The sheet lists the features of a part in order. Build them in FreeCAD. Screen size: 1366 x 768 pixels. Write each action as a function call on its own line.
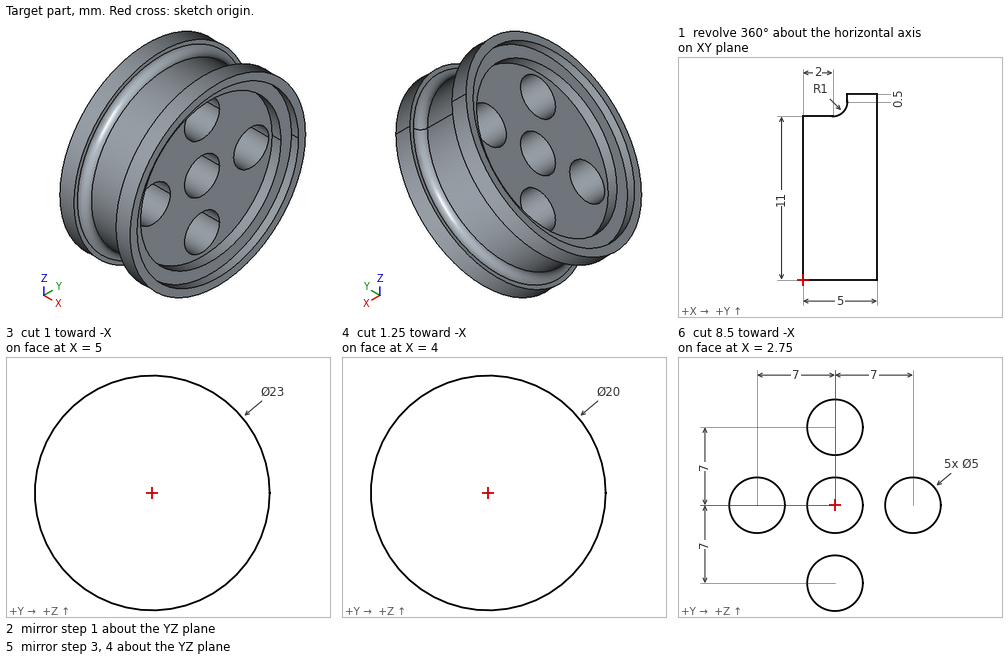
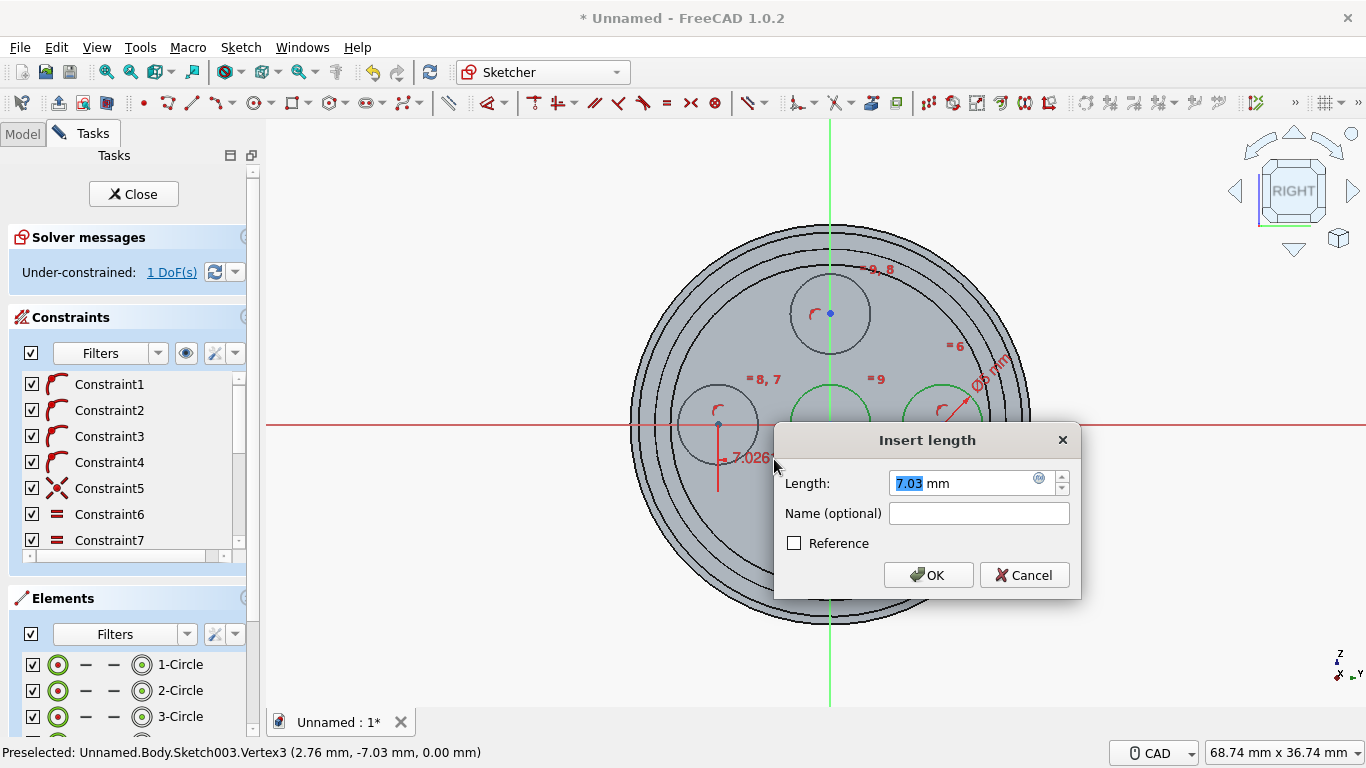
text(7)
key(Return)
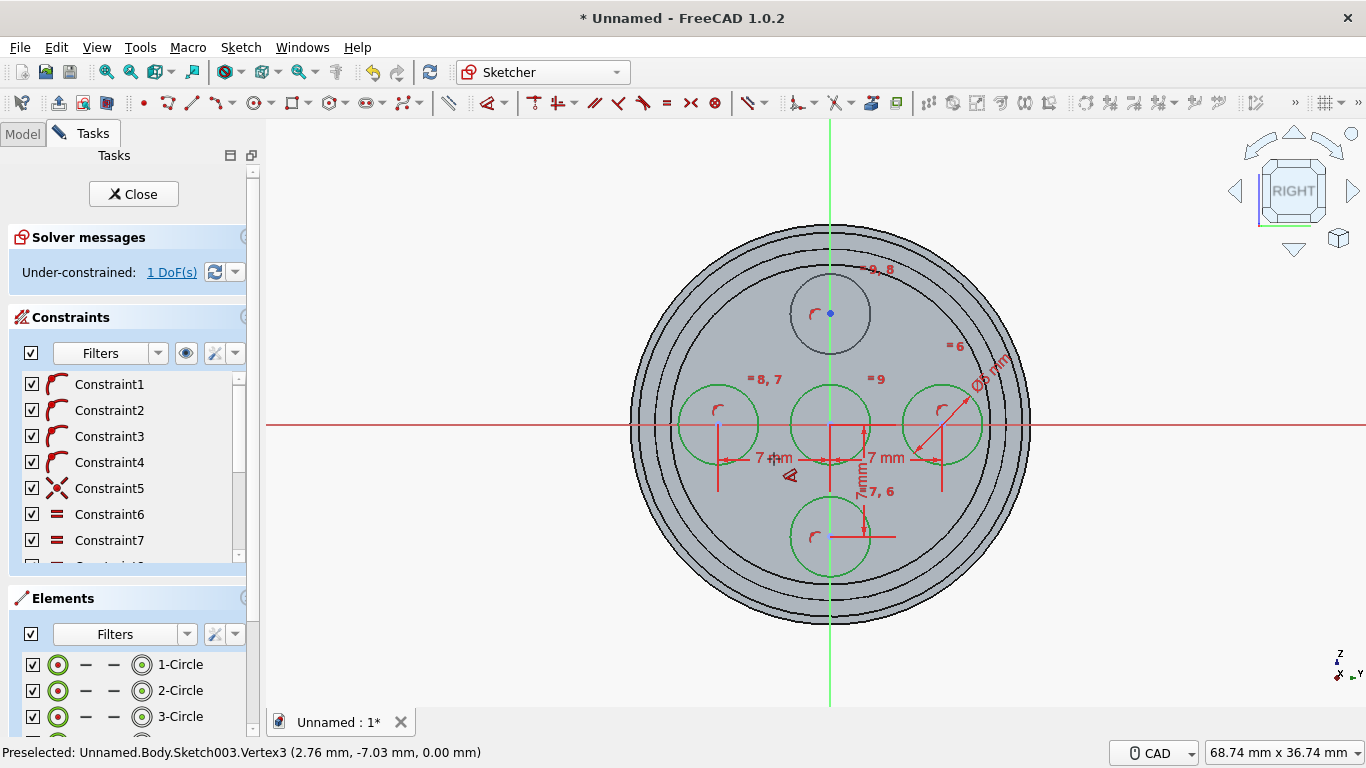
click(830, 314)
click(864, 369)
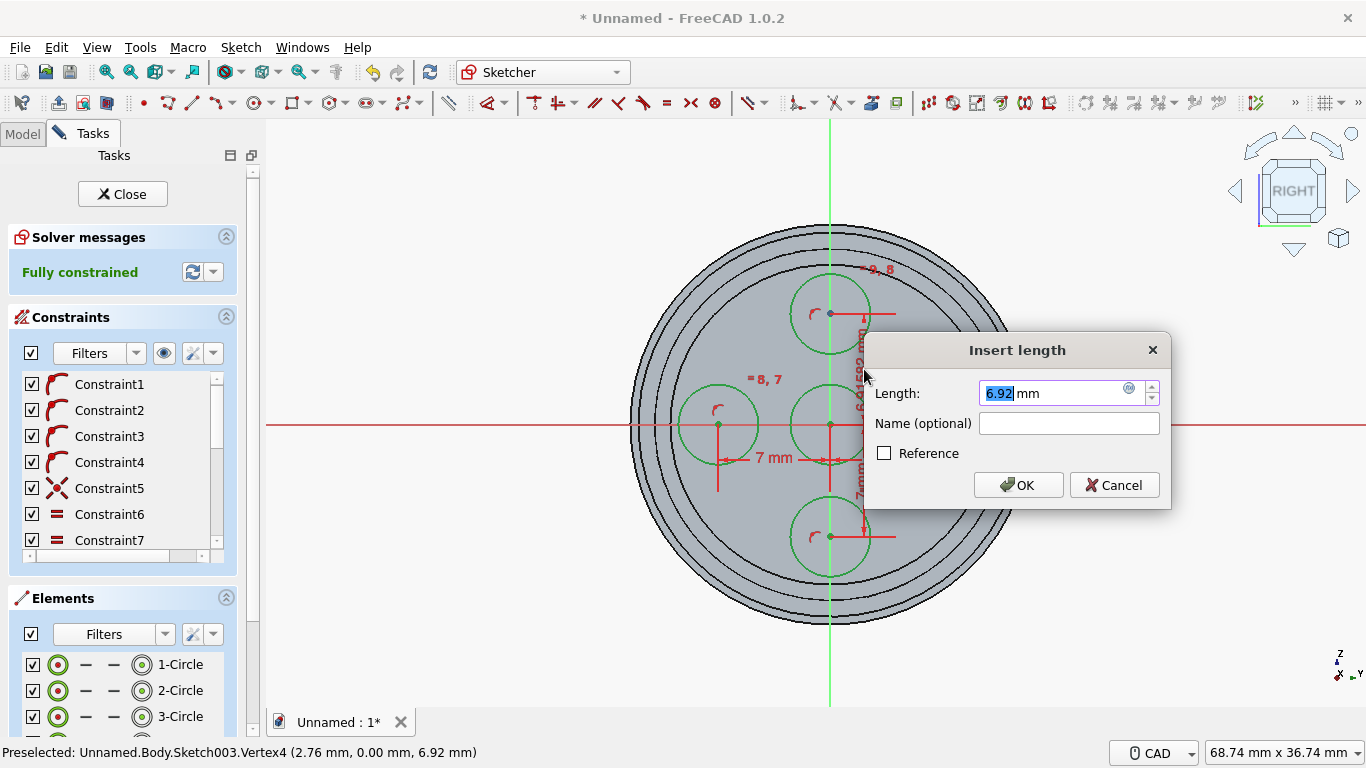
text(7)
key(Return)
key(Escape)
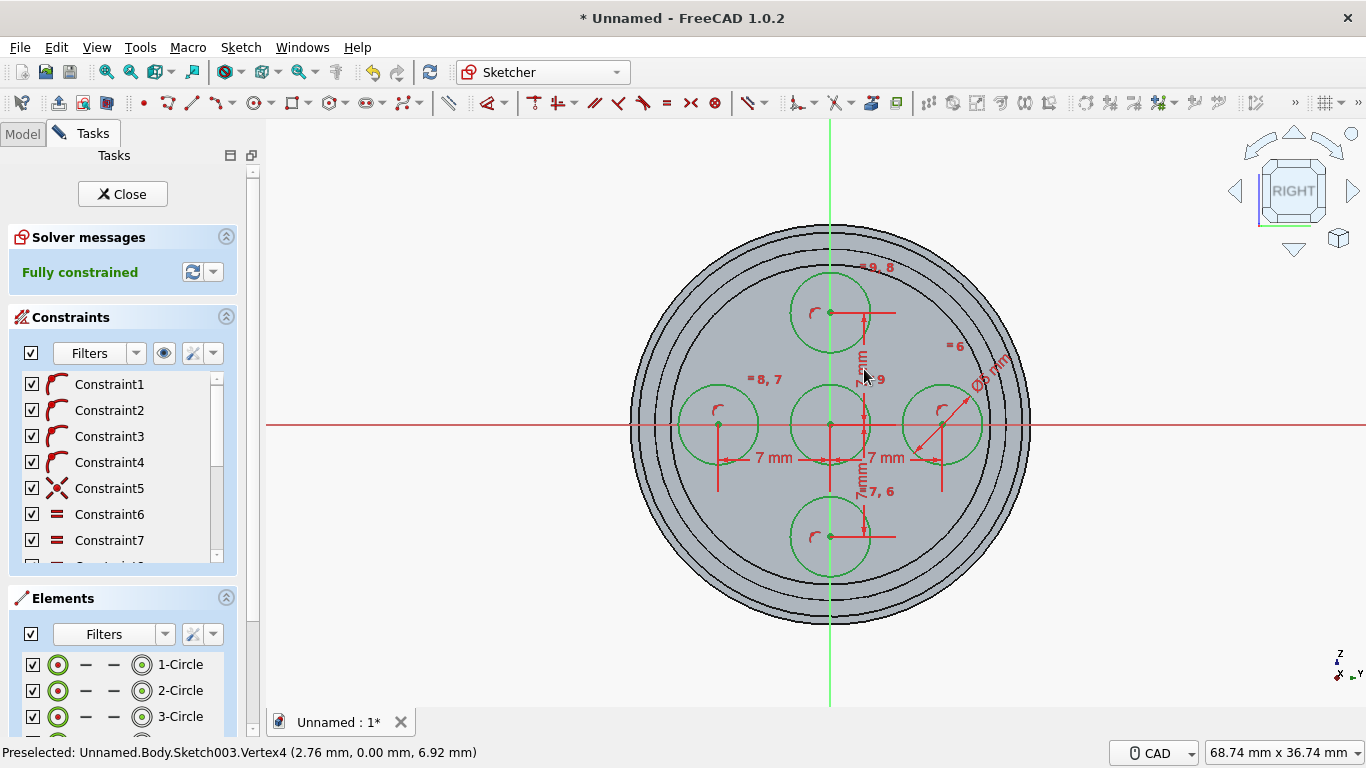
click(123, 194)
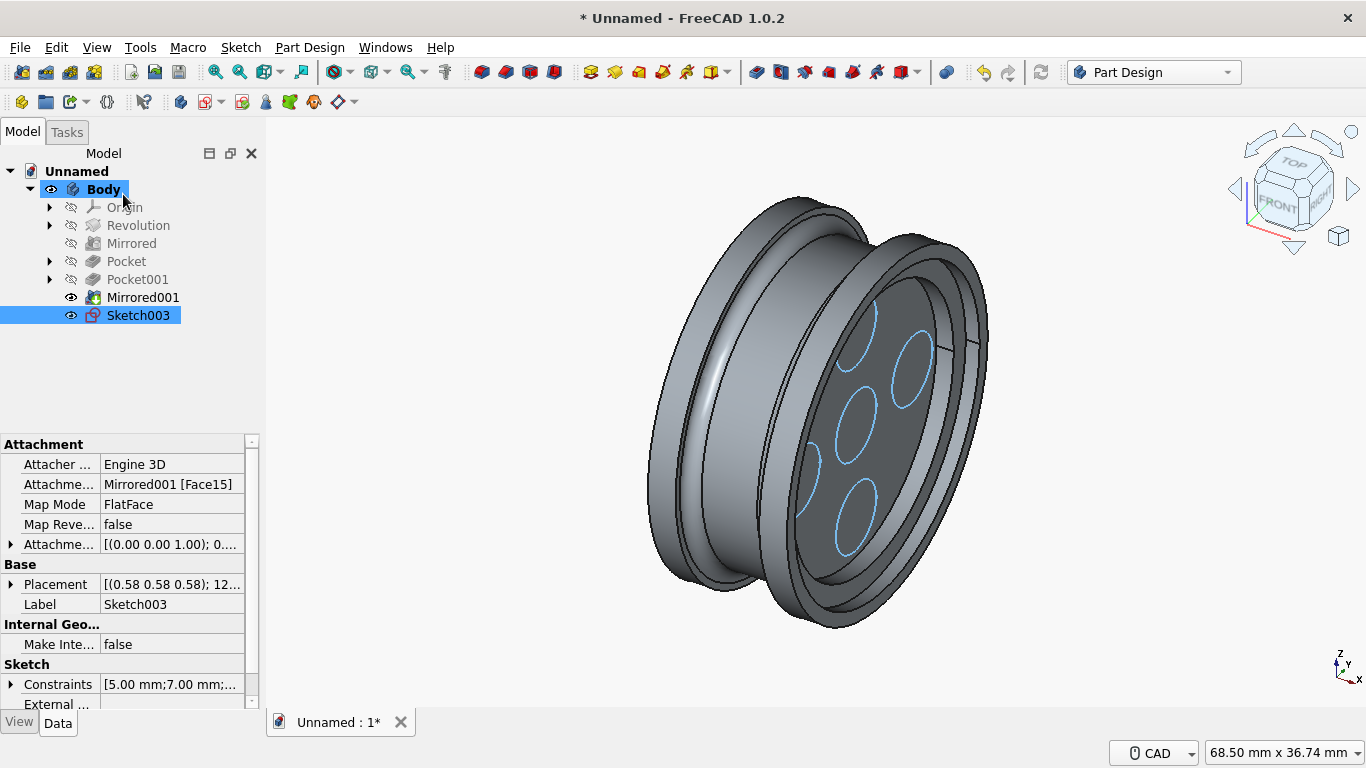
click(758, 72)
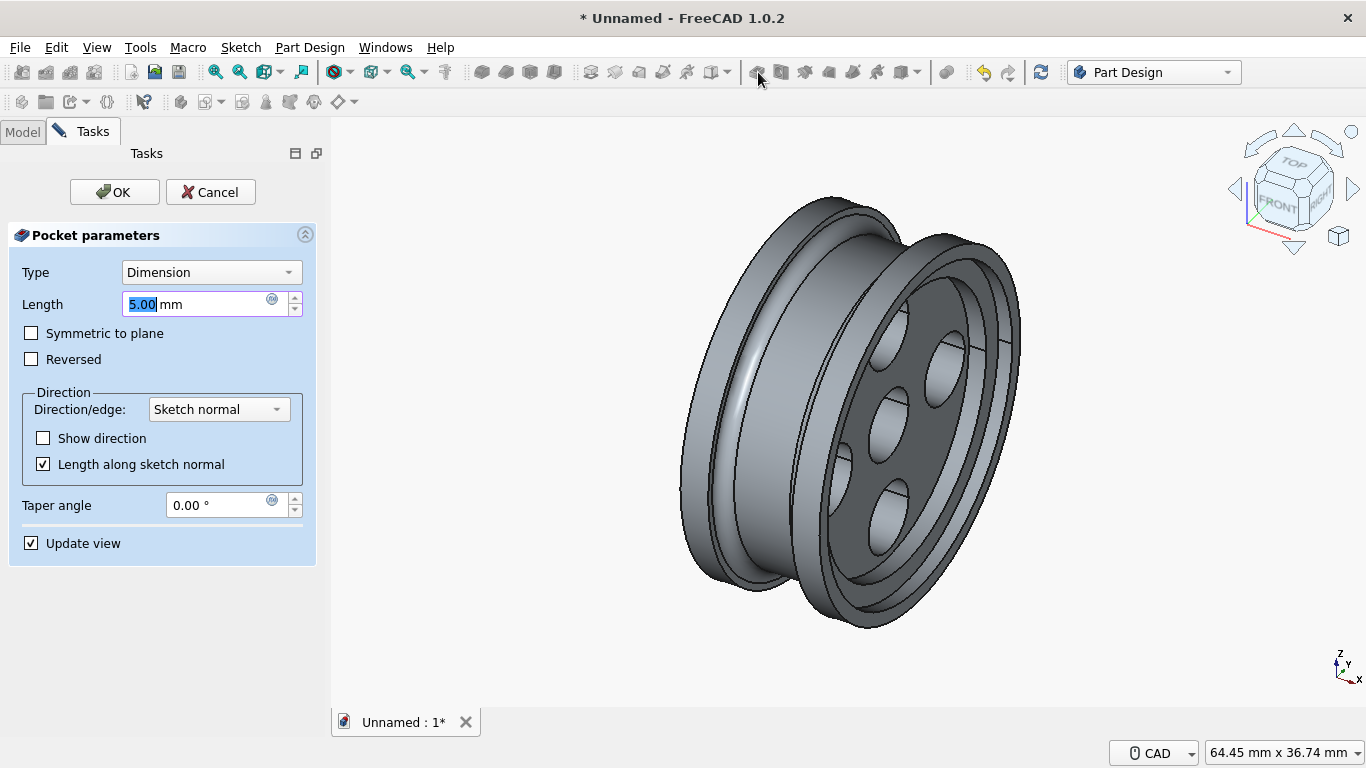
text(8.5)
key(Tab)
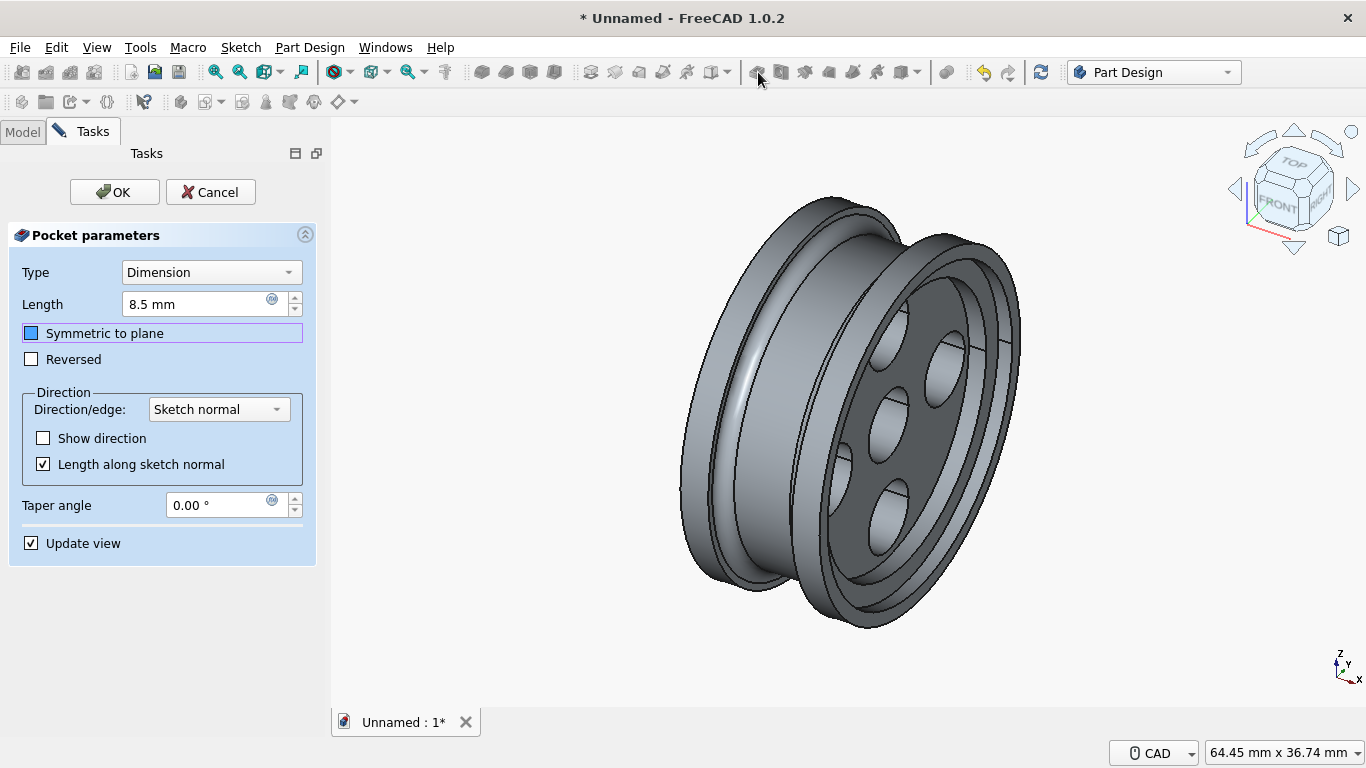
click(115, 192)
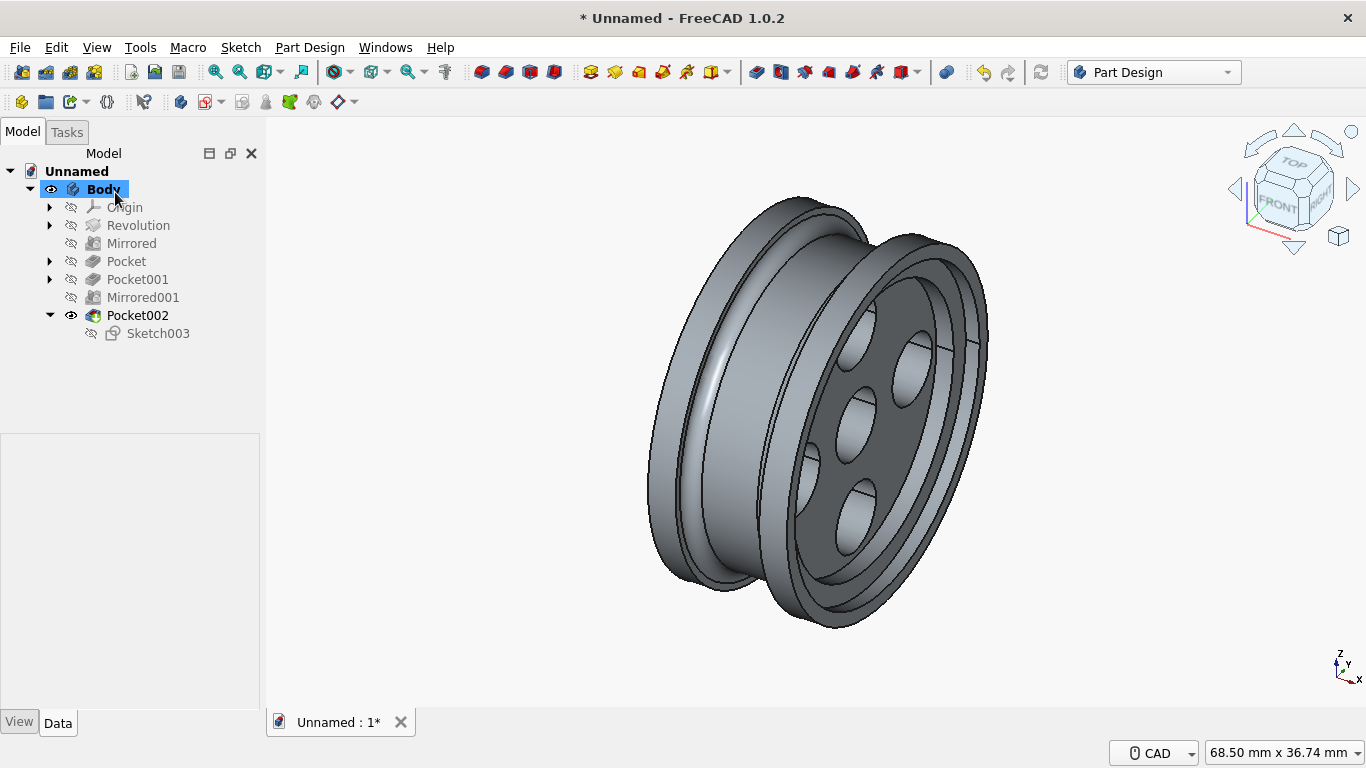
key(0)